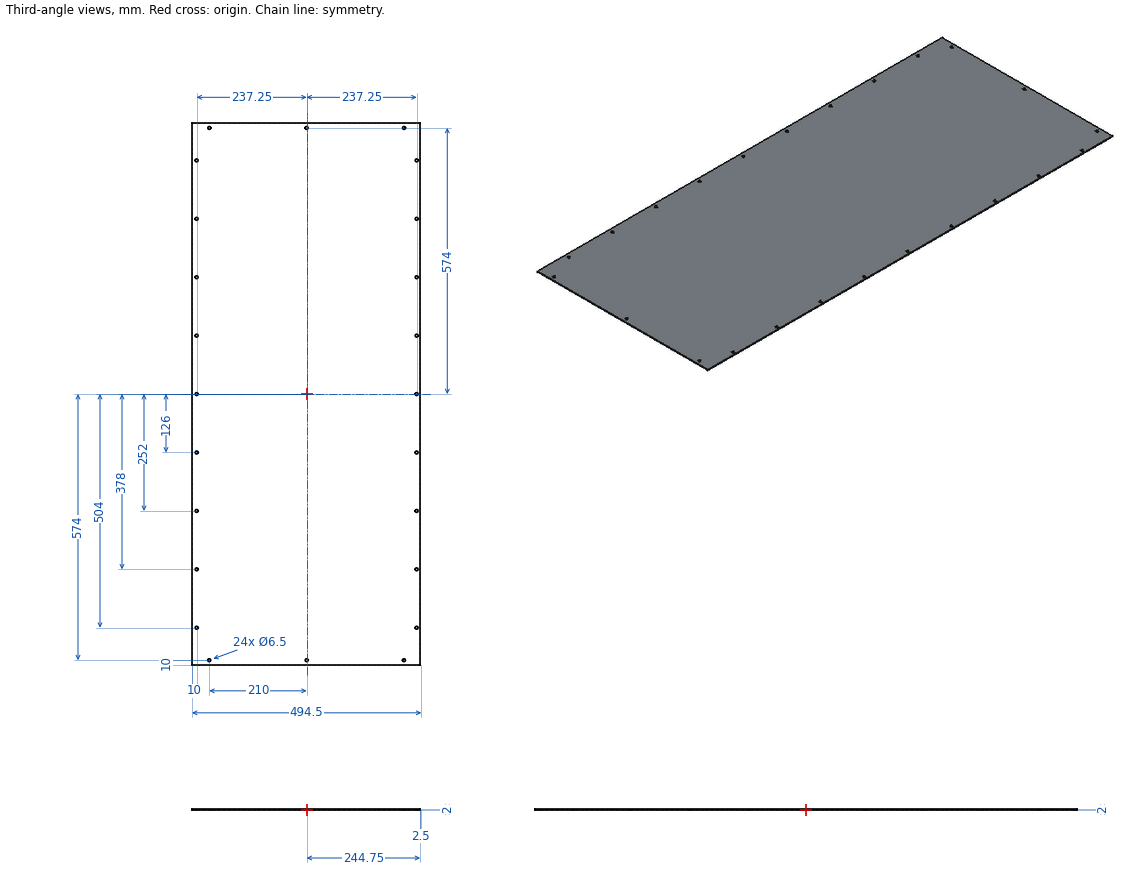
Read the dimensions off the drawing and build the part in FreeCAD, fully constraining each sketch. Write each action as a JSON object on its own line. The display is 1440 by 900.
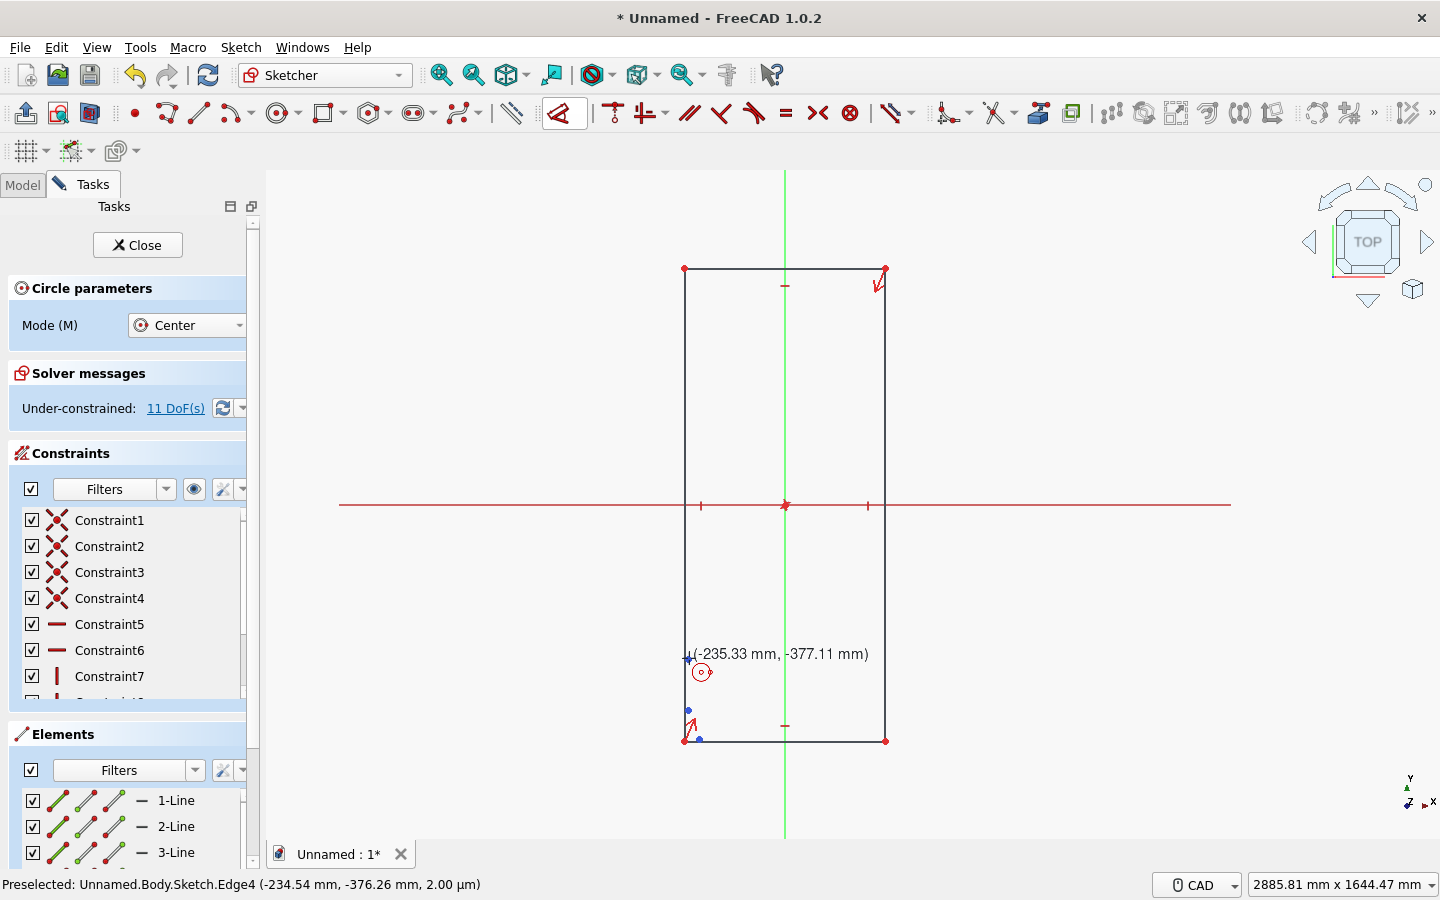
{"action": "scroll", "coordinate": [689, 608], "scroll_direction": "up", "scroll_amount": 15}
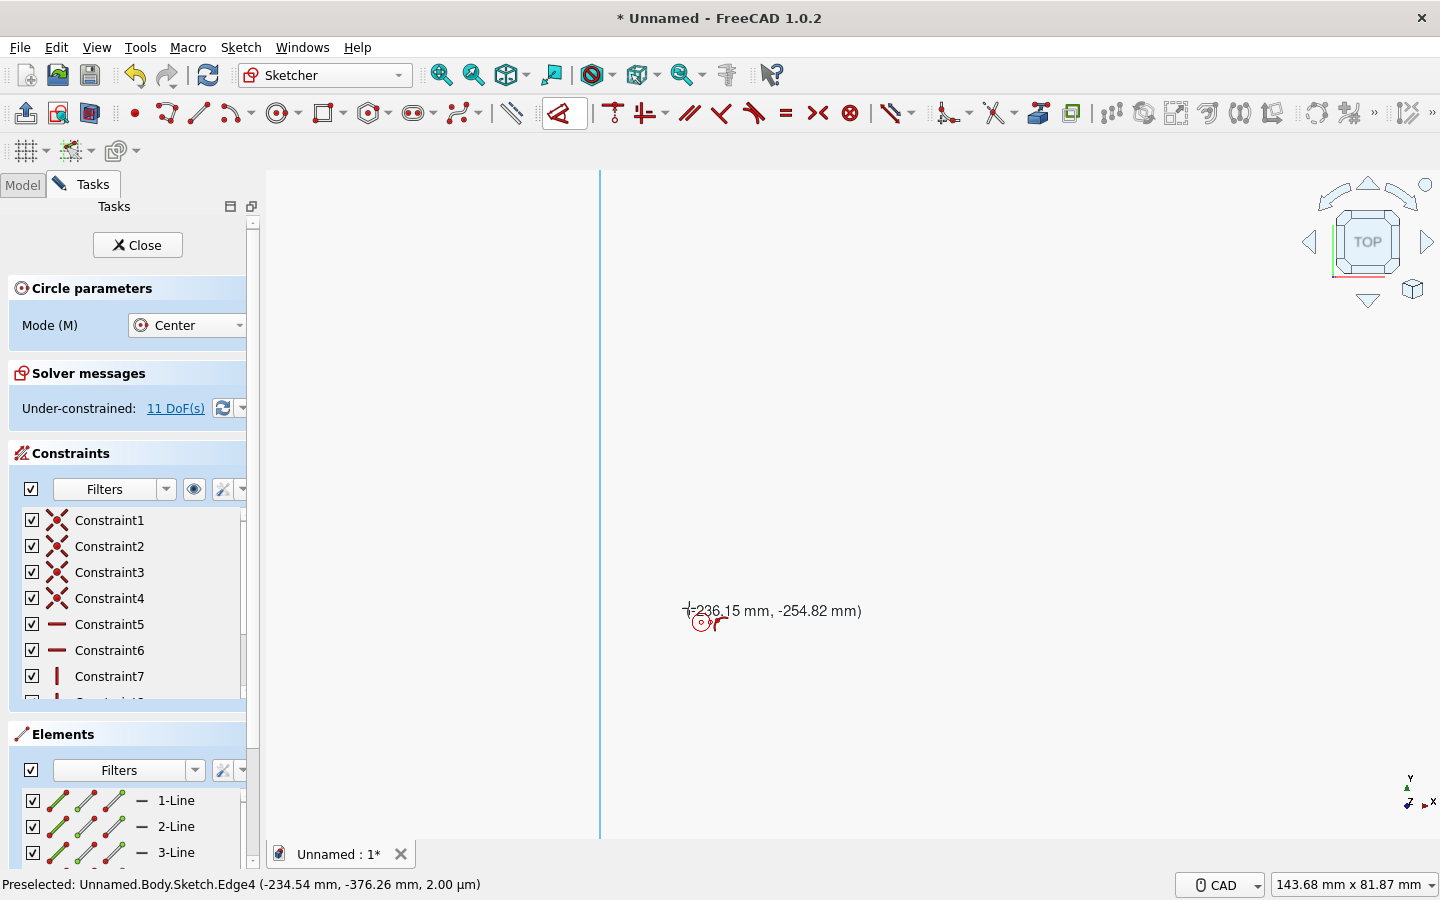
{"action": "scroll", "coordinate": [689, 608], "scroll_direction": "down", "scroll_amount": 15}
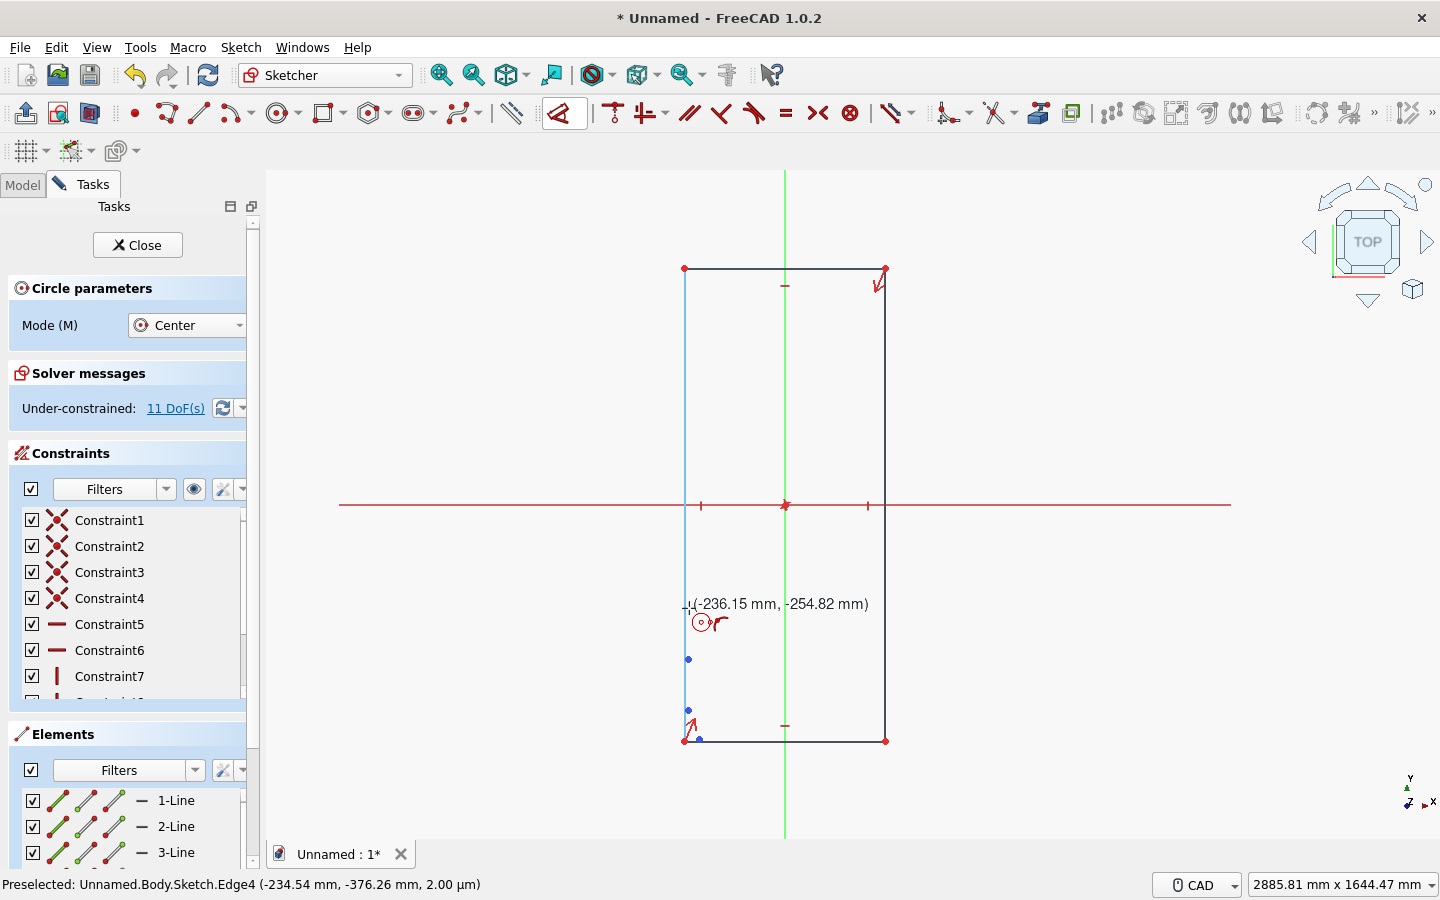
{"action": "scroll", "coordinate": [689, 608], "scroll_direction": "up", "scroll_amount": 7}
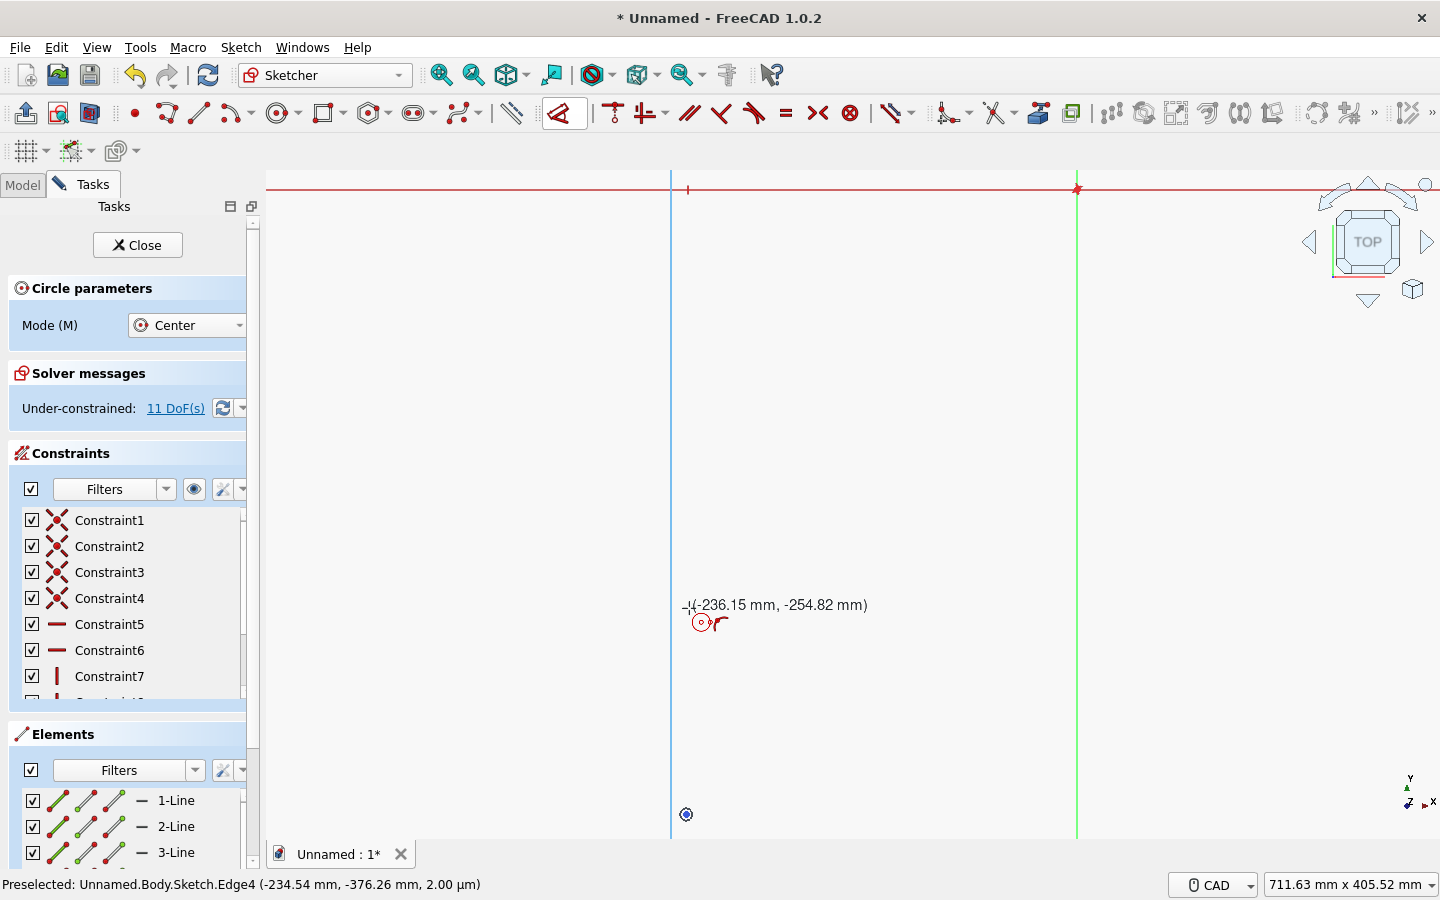
{"action": "left_click", "coordinate": [686, 605]}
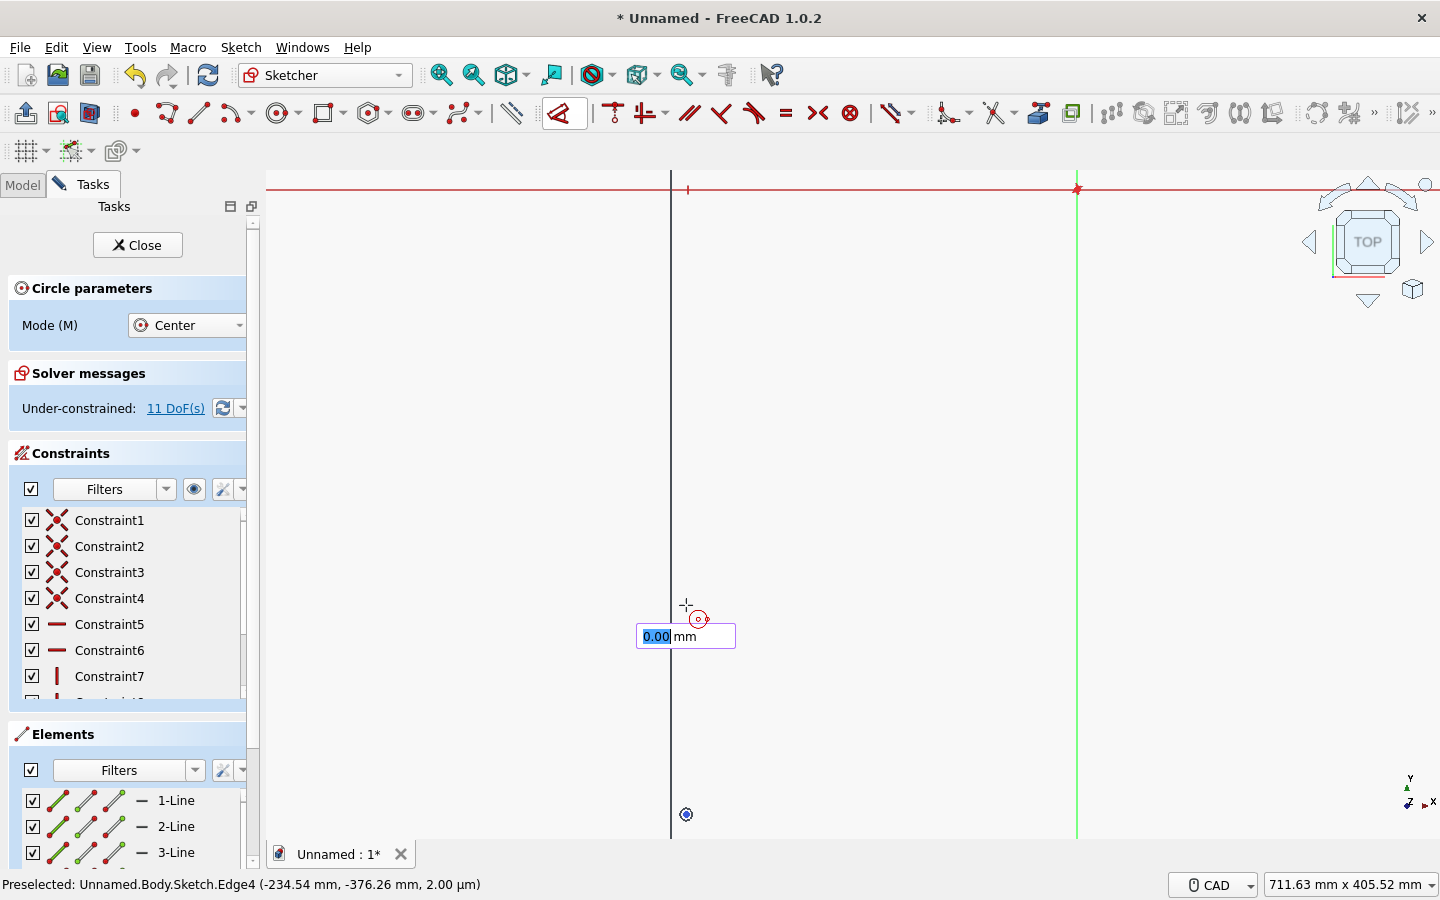
{"action": "scroll", "coordinate": [690, 602], "scroll_direction": "up", "scroll_amount": 6}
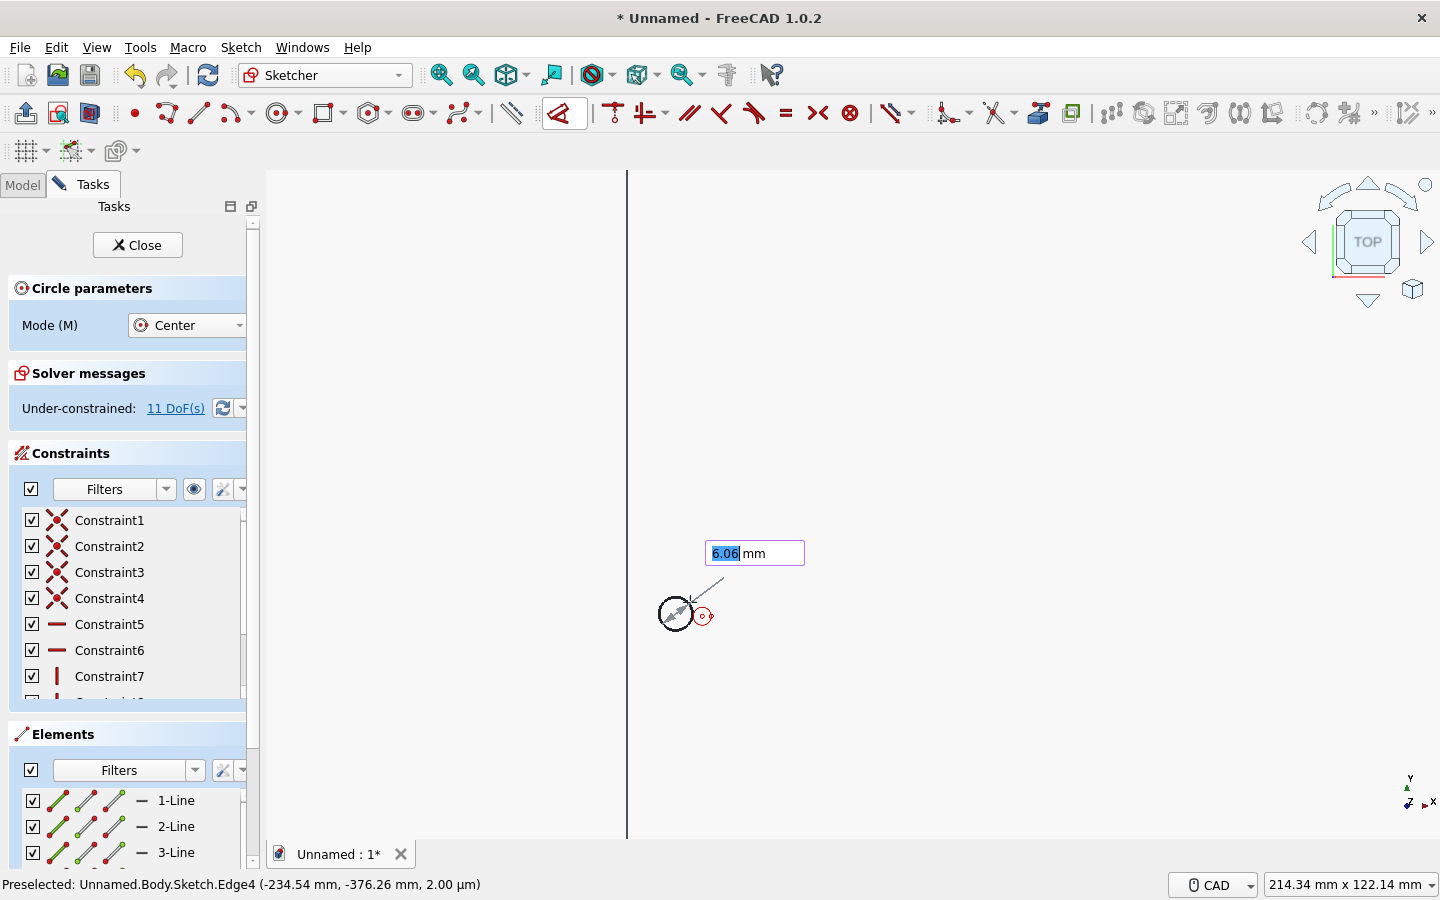
{"action": "left_click", "coordinate": [689, 599]}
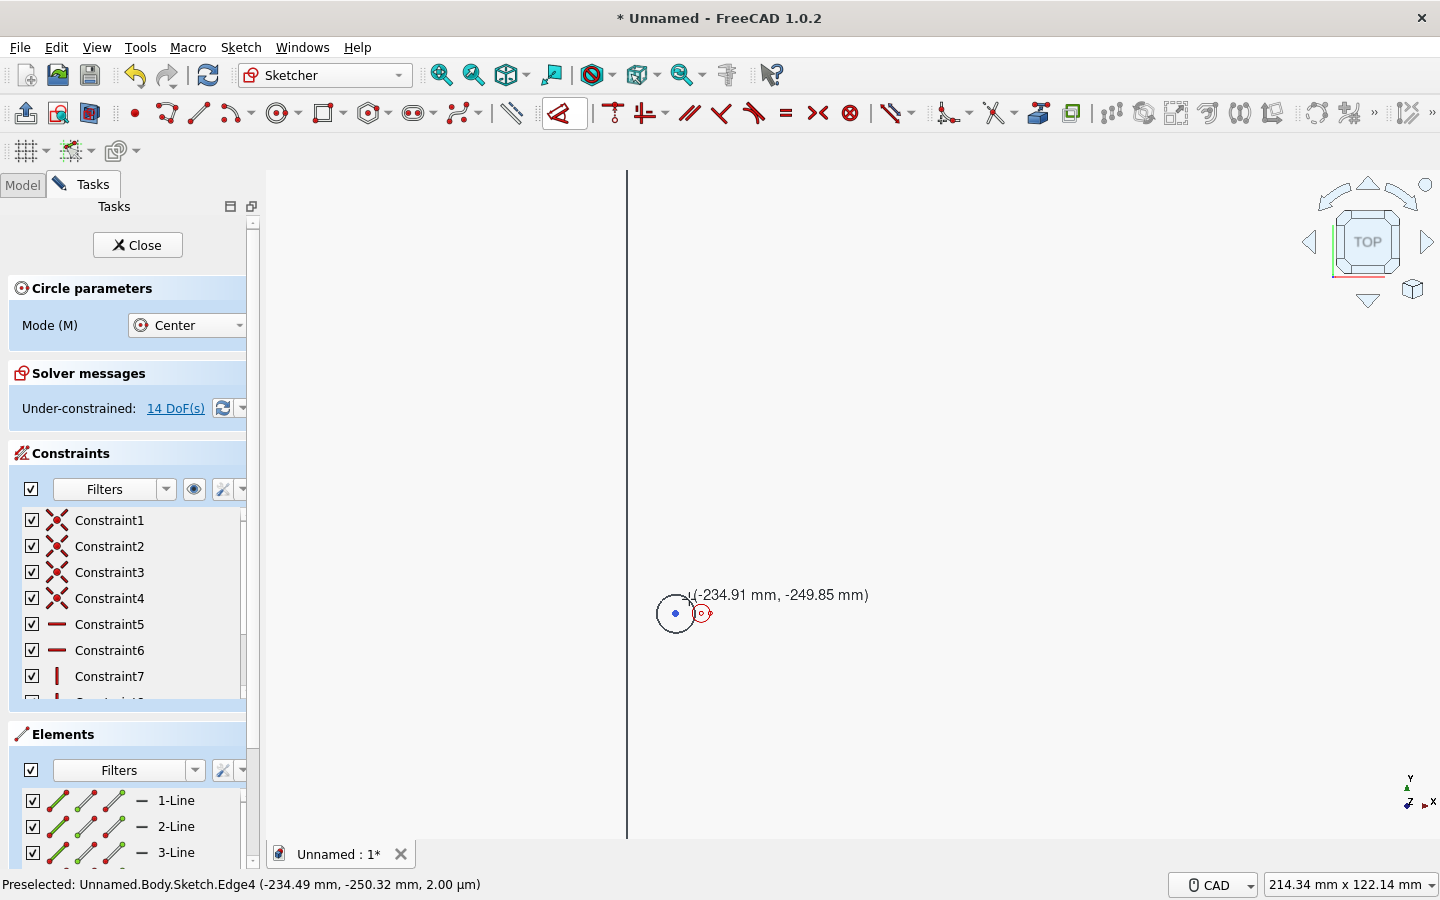
{"action": "scroll", "coordinate": [689, 607], "scroll_direction": "down", "scroll_amount": 13}